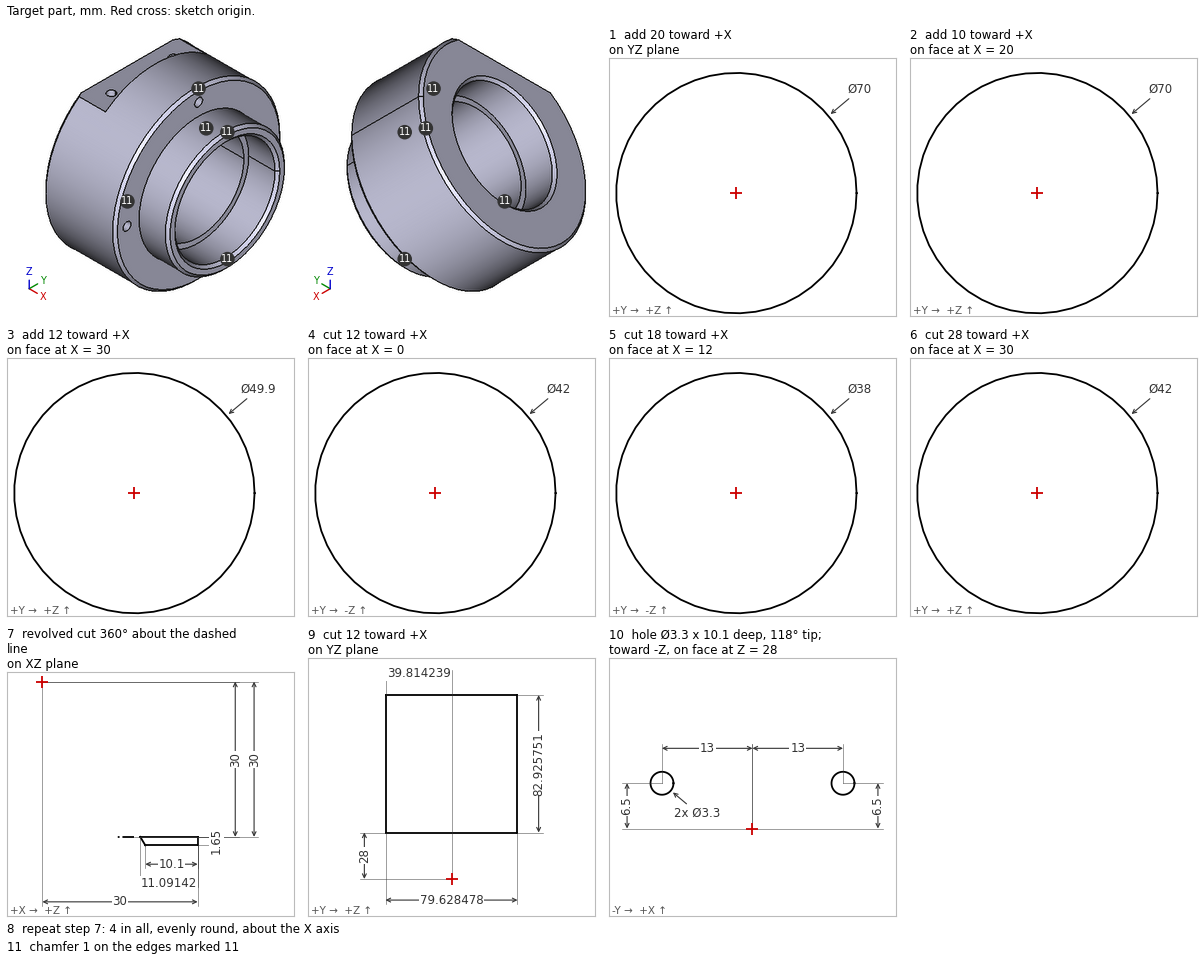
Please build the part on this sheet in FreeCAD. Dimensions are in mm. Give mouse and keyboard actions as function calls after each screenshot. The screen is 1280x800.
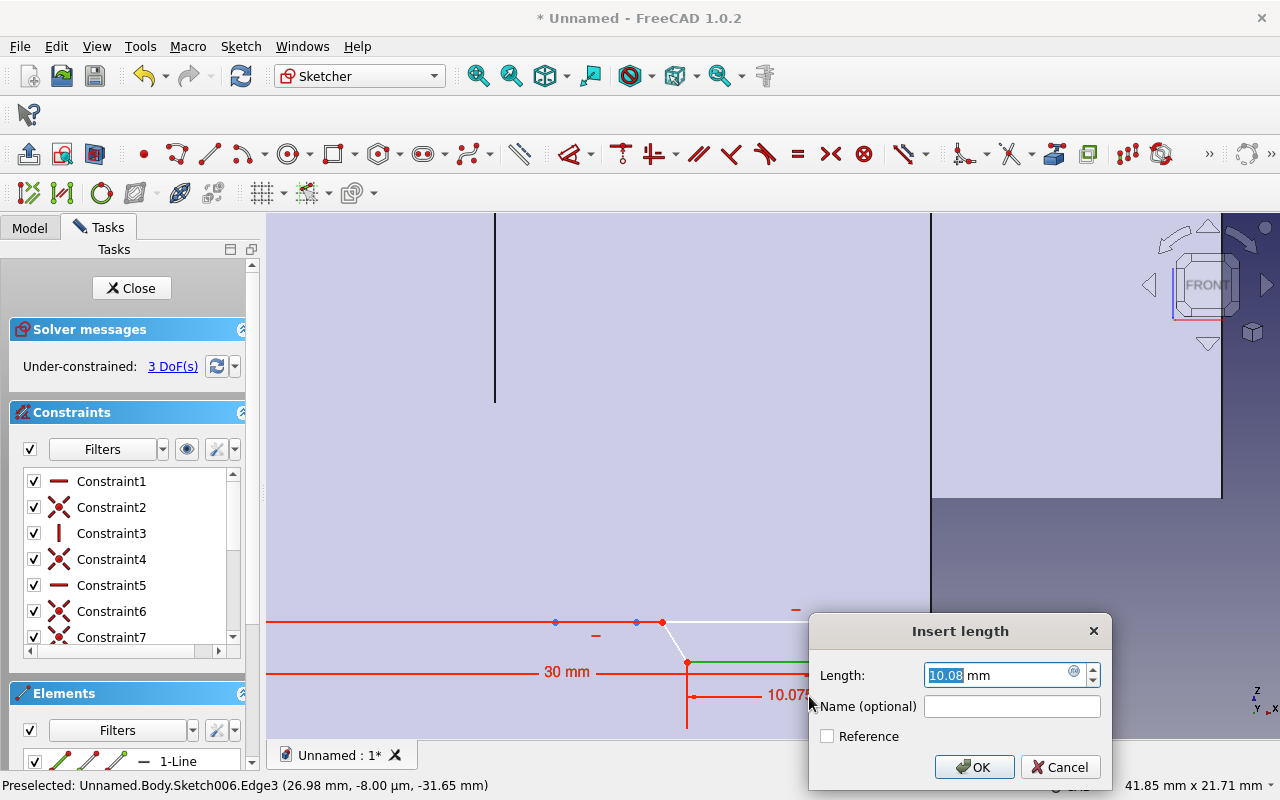
text(10.1)
key(Return)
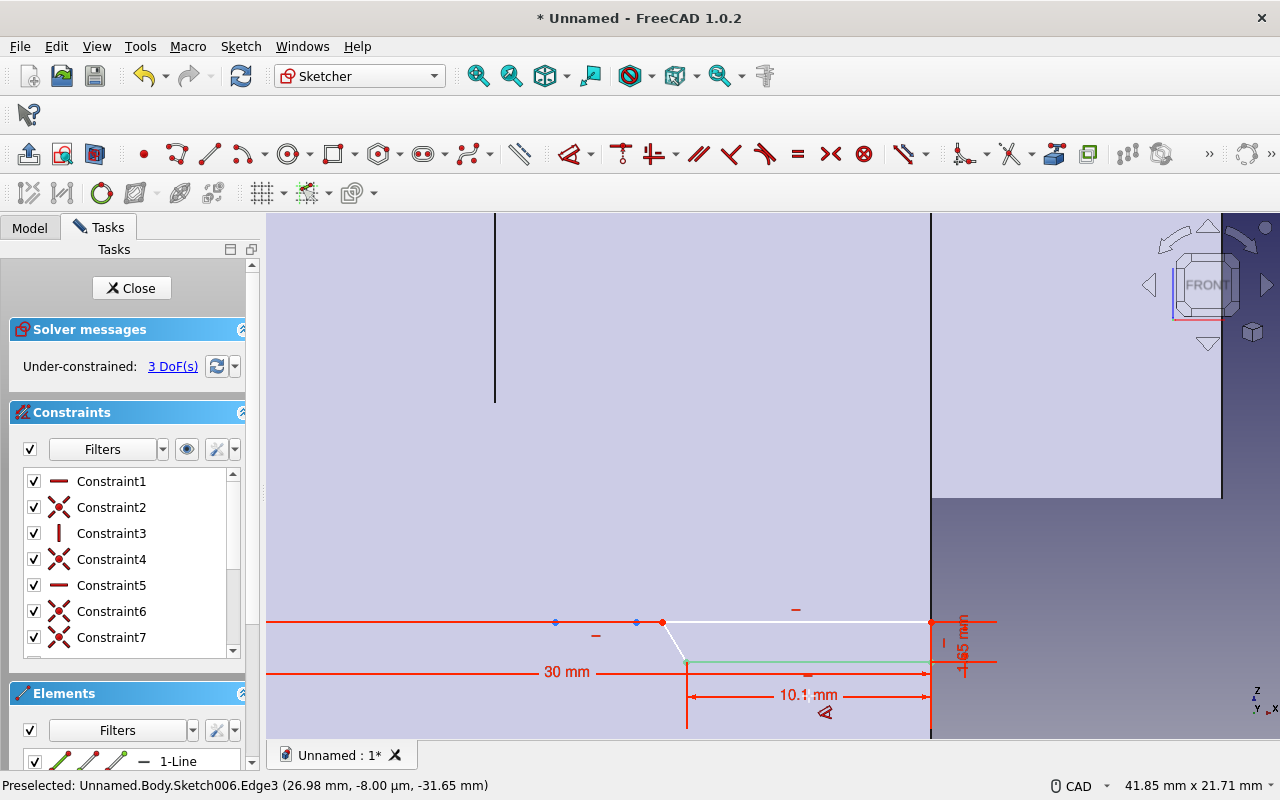
click(743, 622)
click(797, 588)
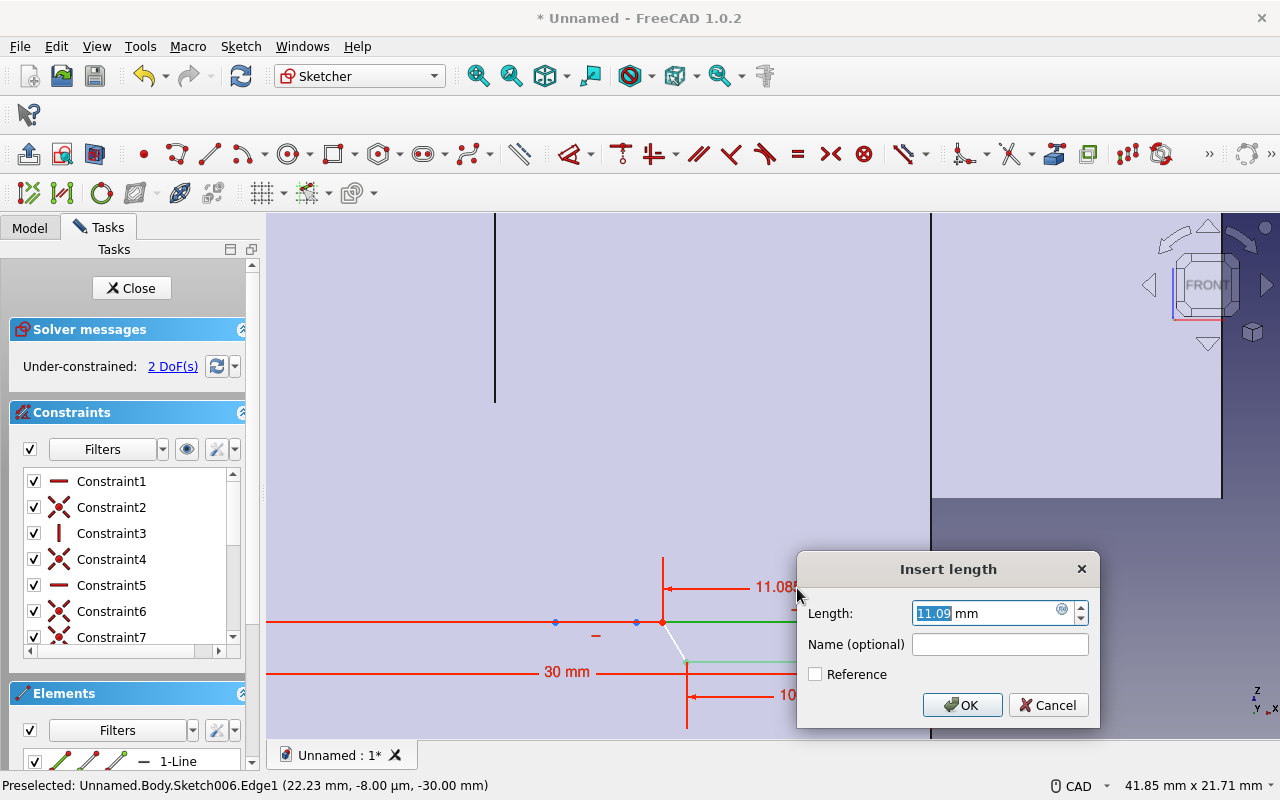
text(11.09142)
key(Return)
key(Escape)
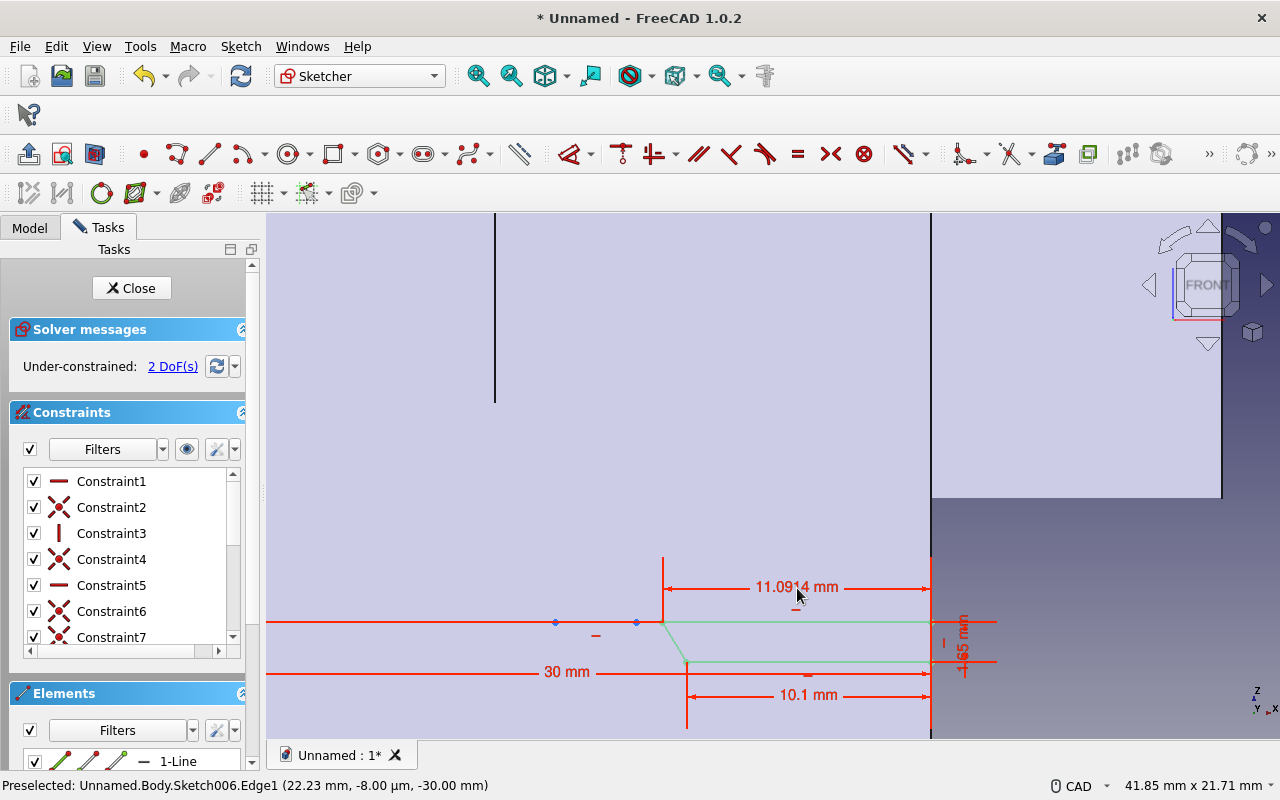
click(132, 288)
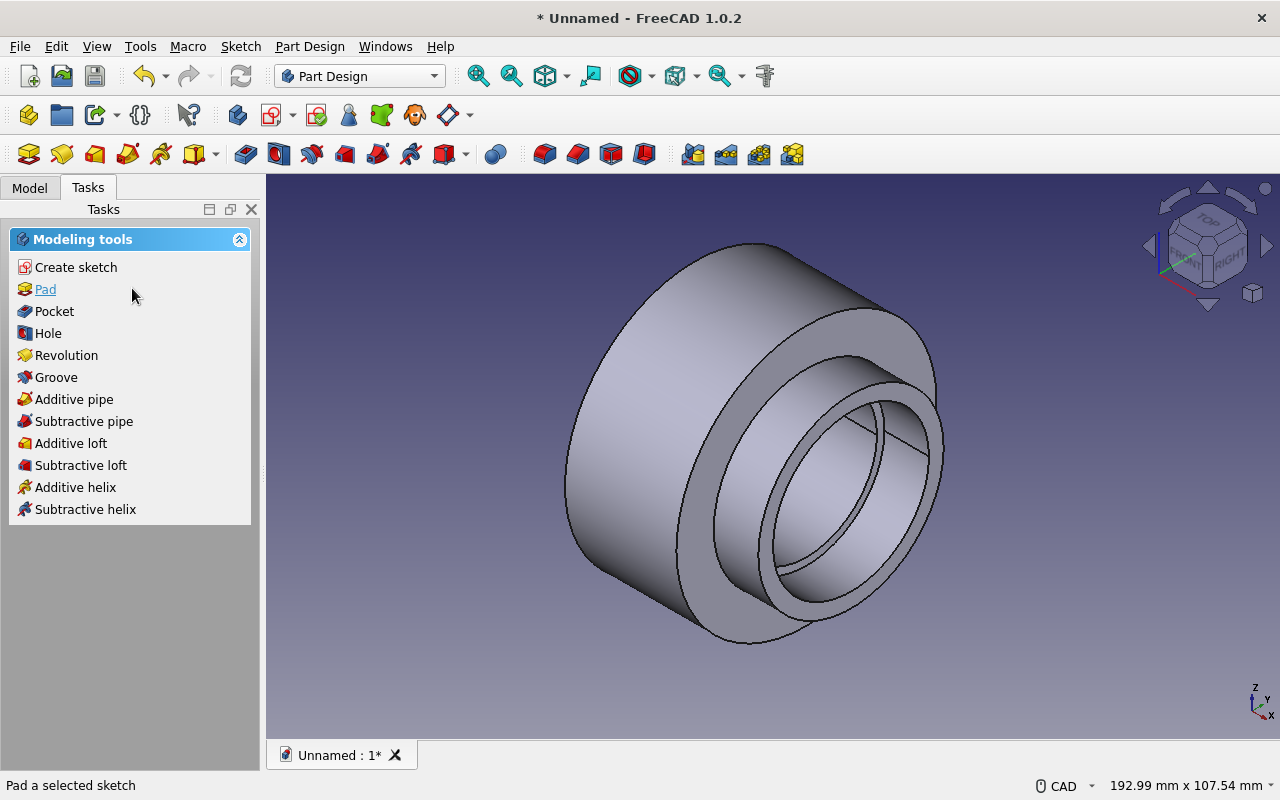
click(312, 154)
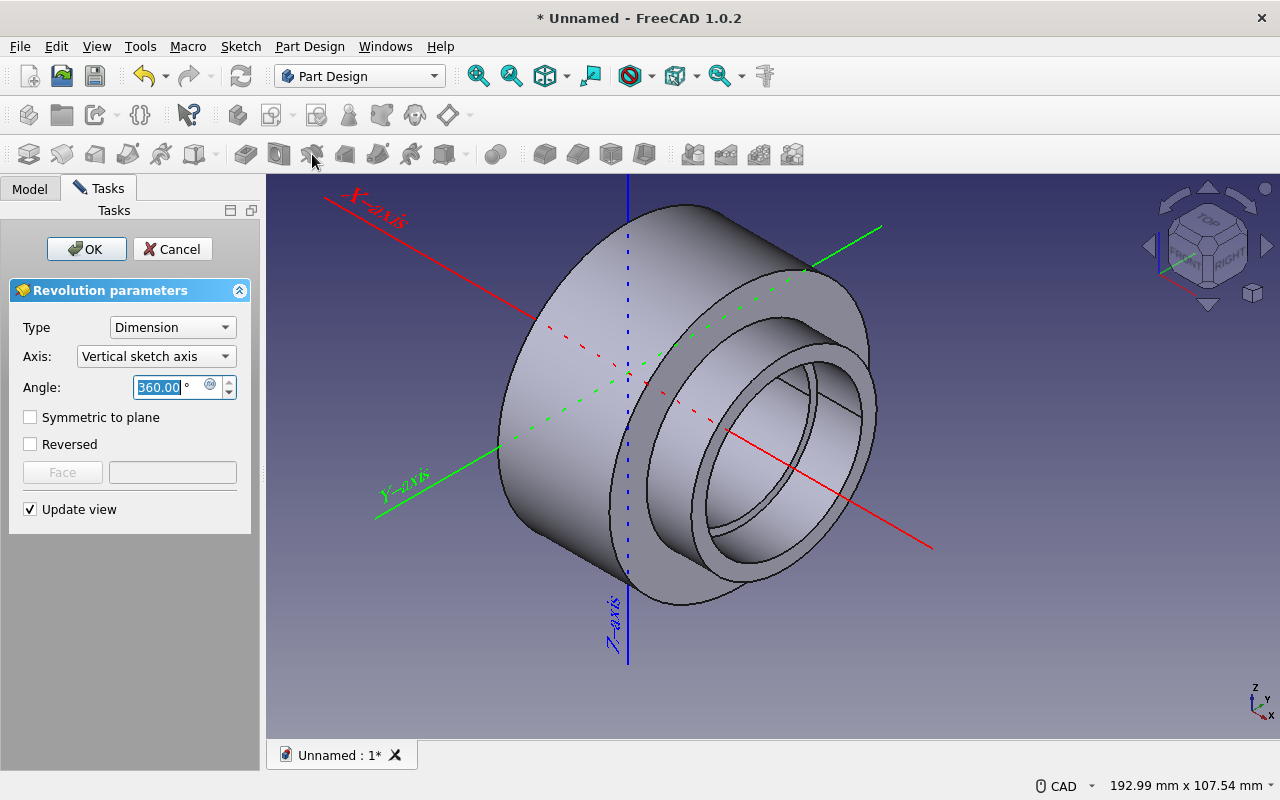
click(157, 356)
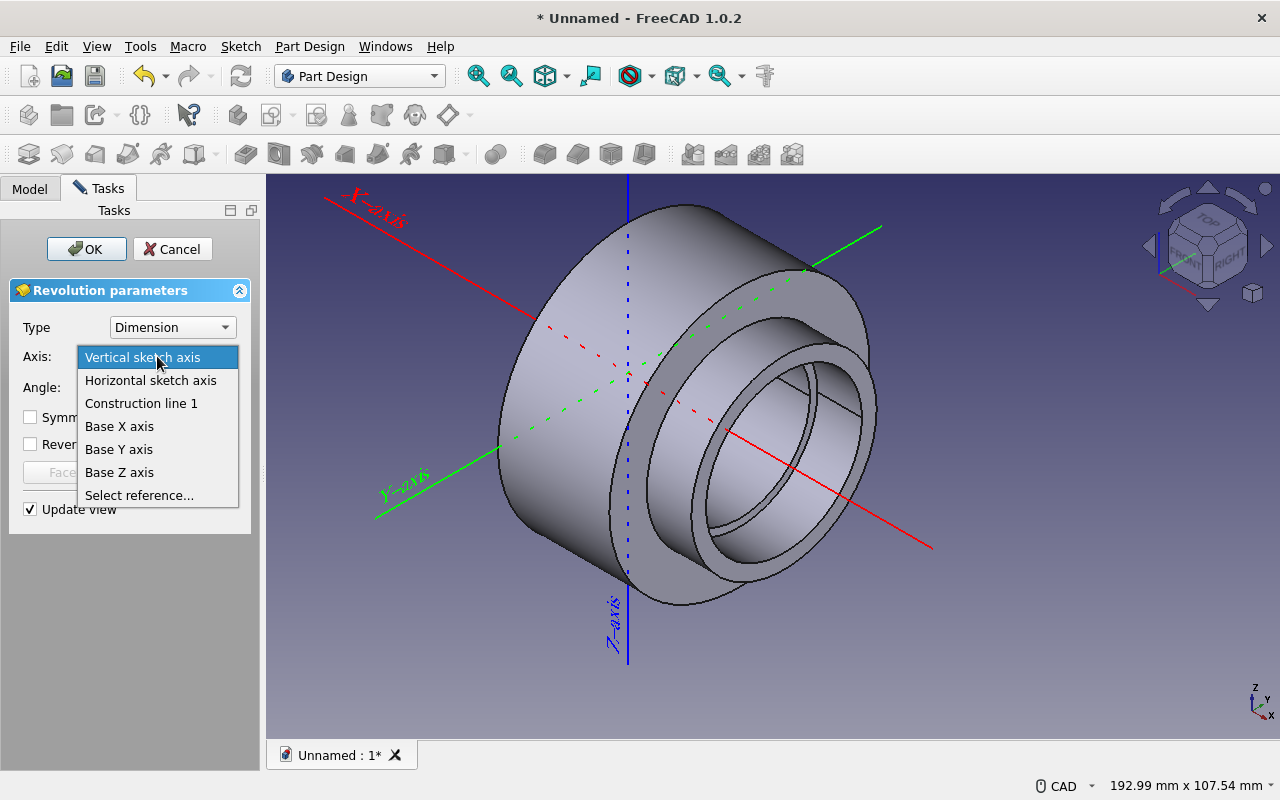
click(156, 404)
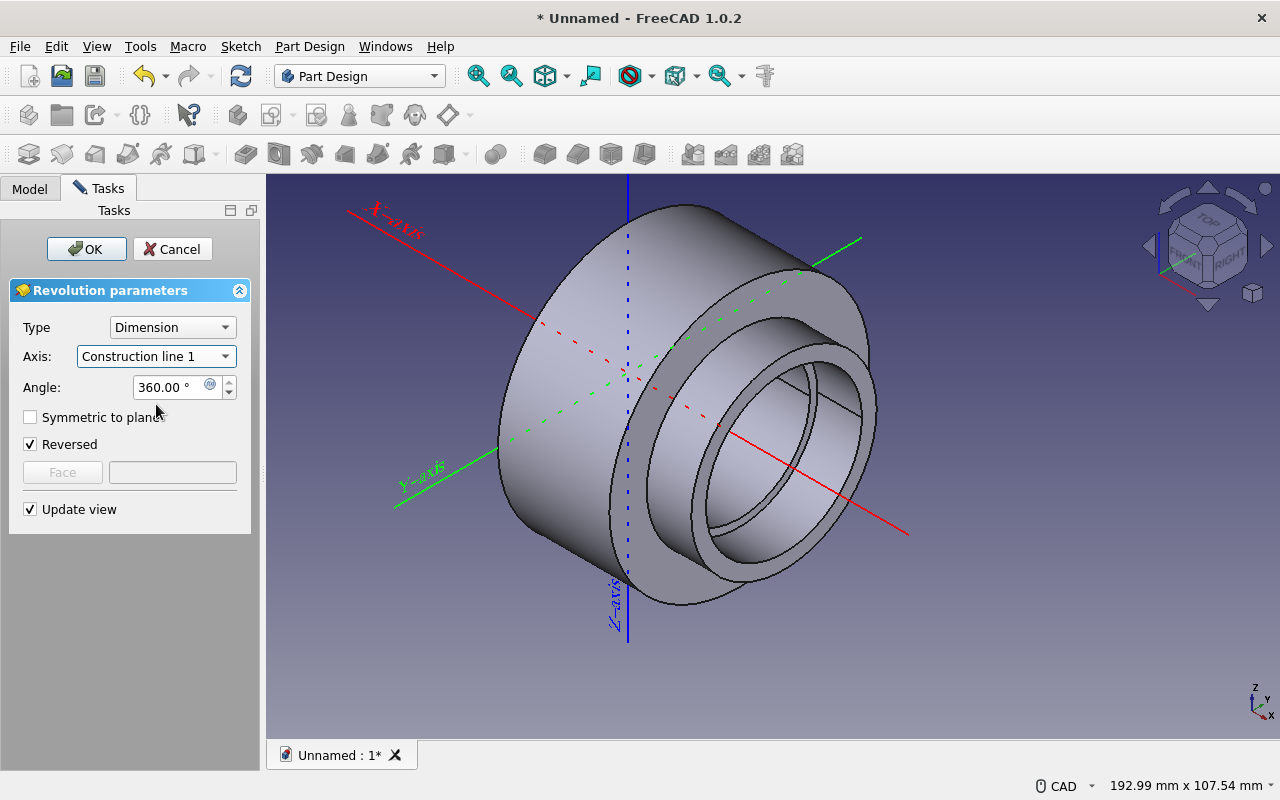
click(87, 249)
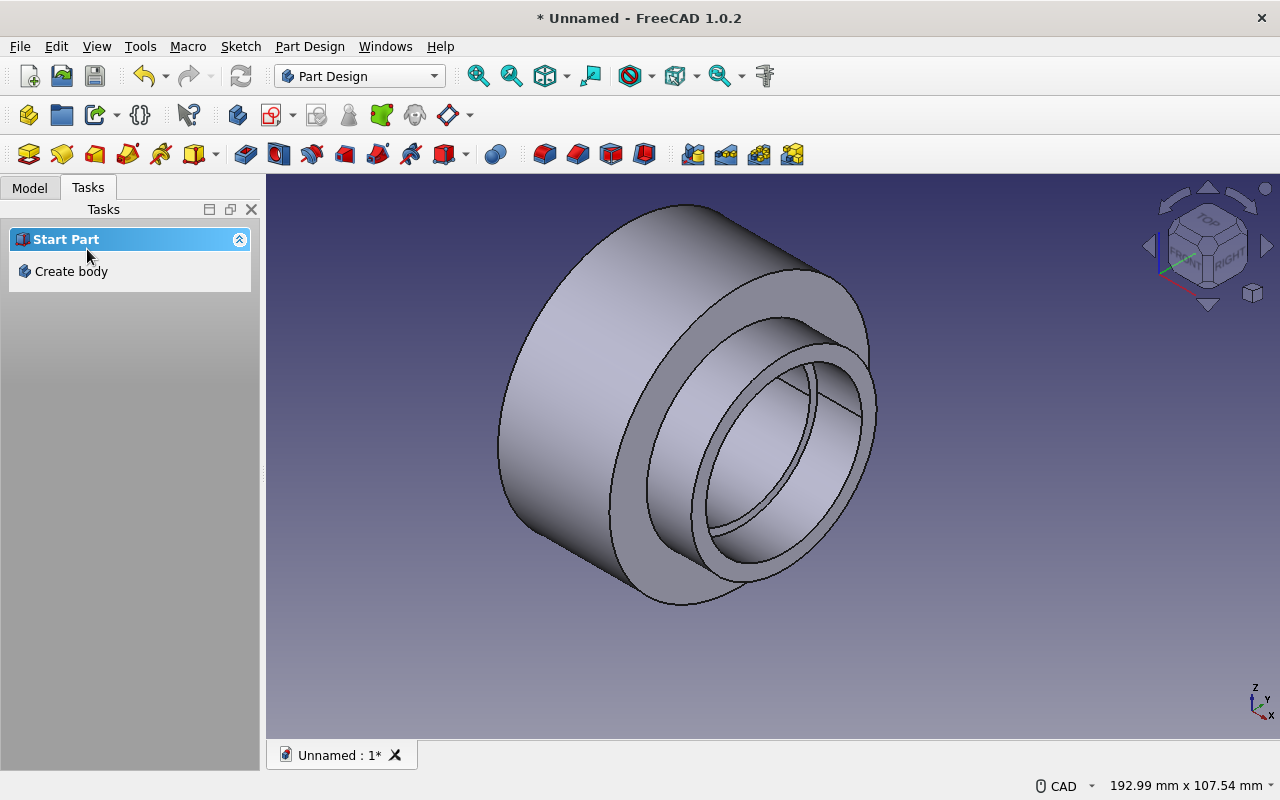
key(v)
key(f)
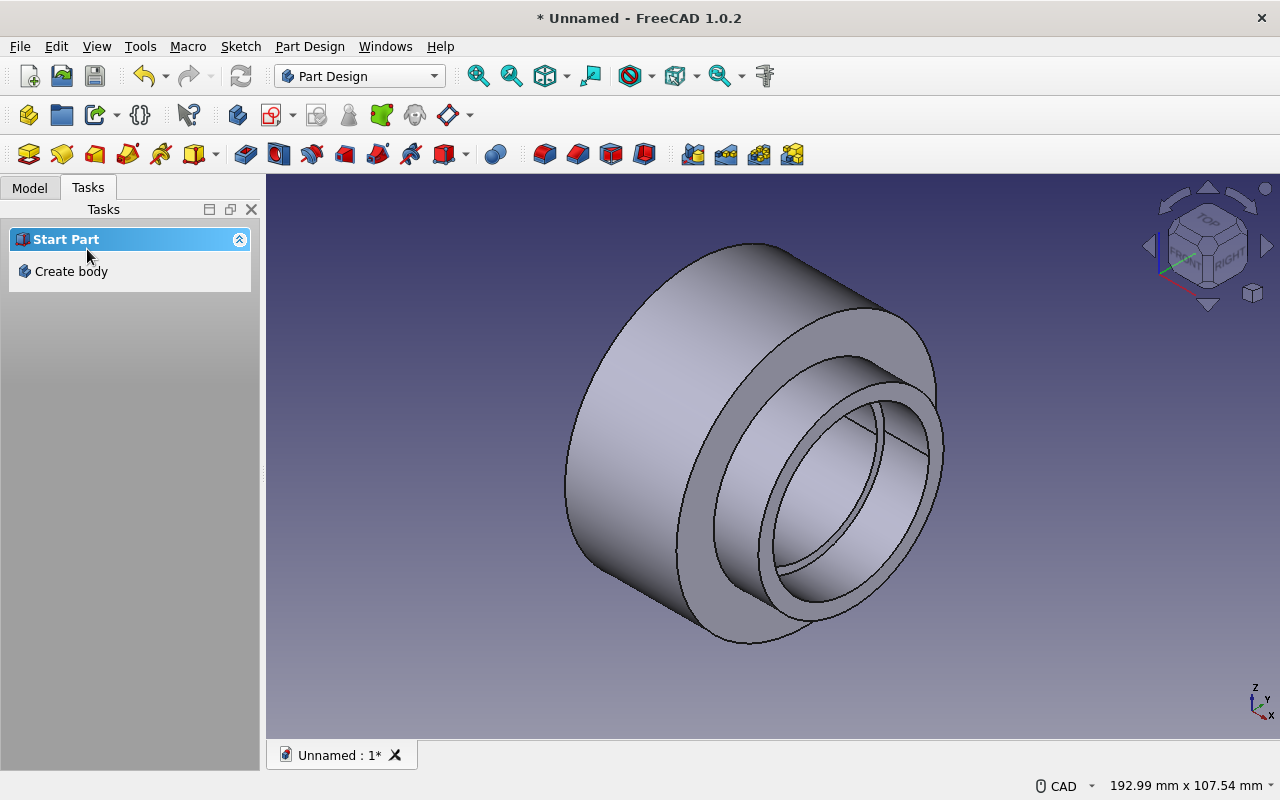
click(30, 188)